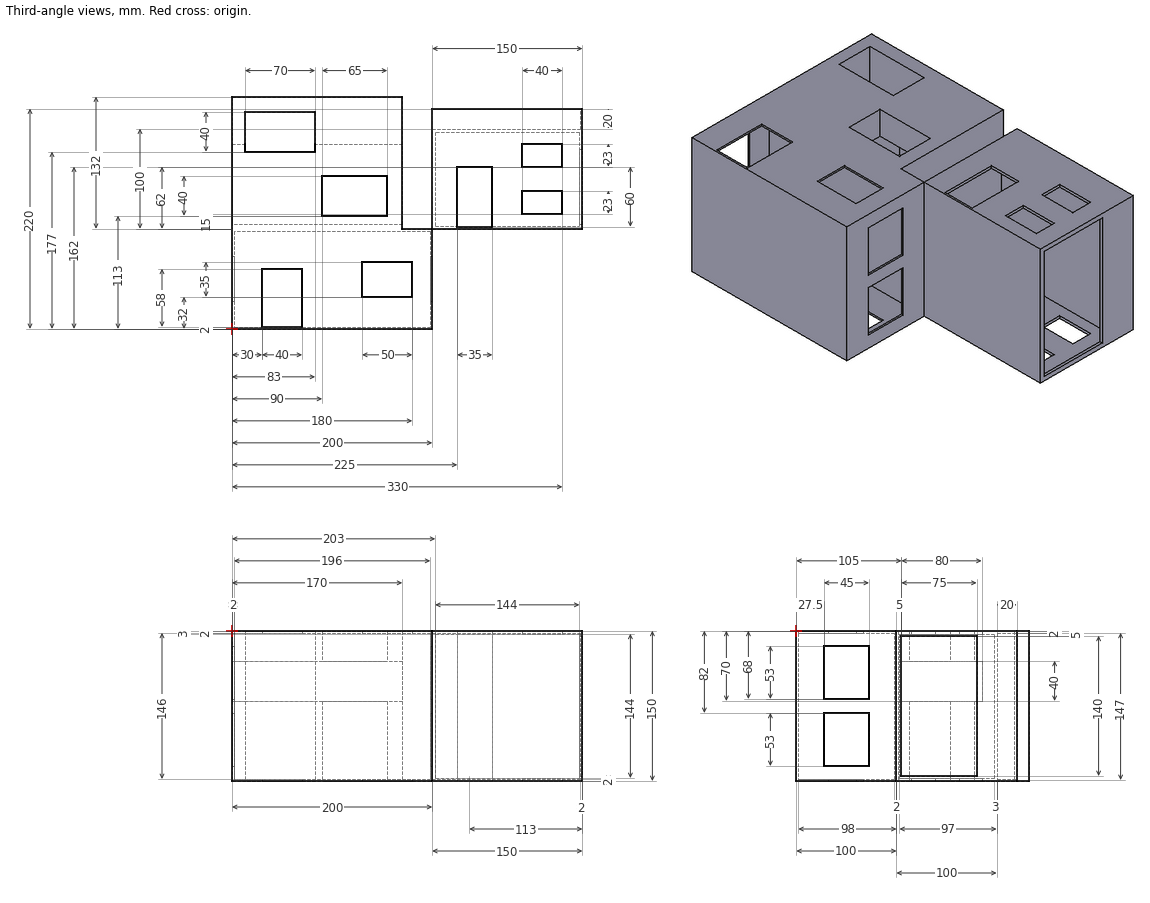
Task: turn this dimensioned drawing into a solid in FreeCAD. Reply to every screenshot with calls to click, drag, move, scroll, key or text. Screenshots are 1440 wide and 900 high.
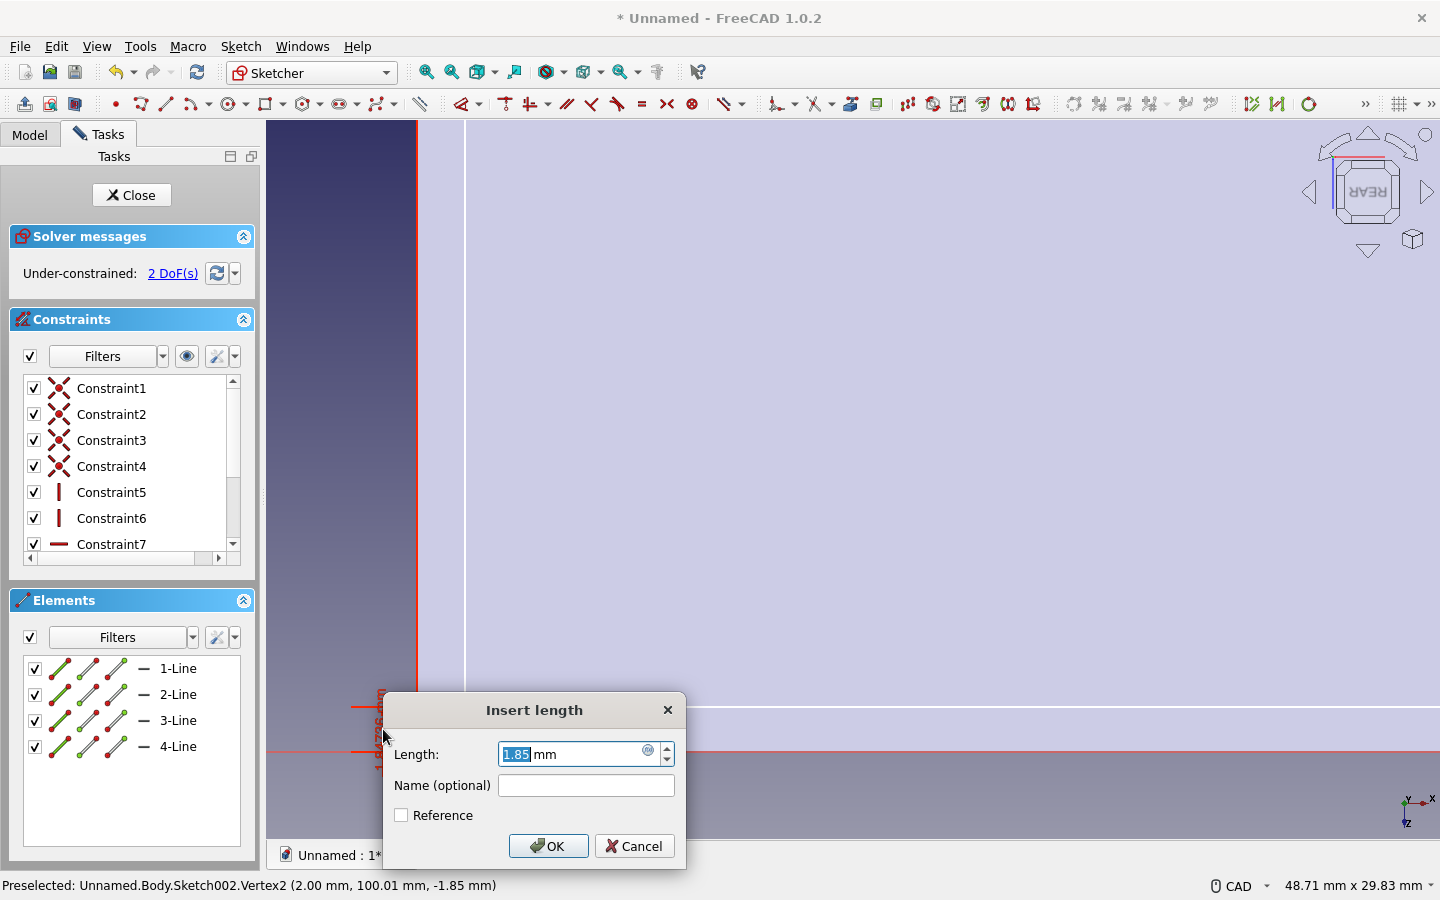
text(2)
key(Return)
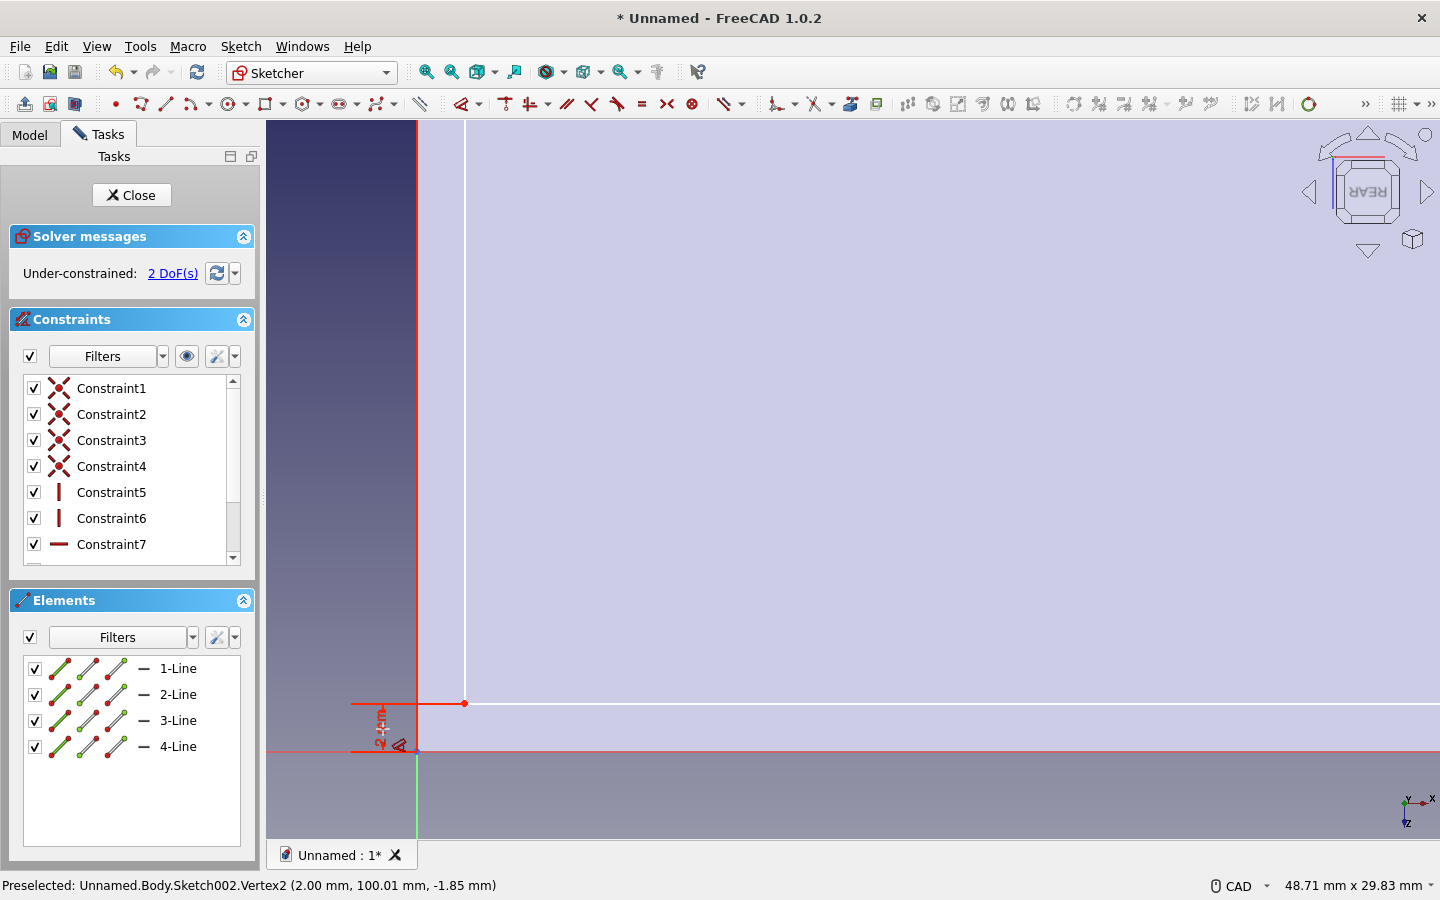
scroll(469, 716, down, 10)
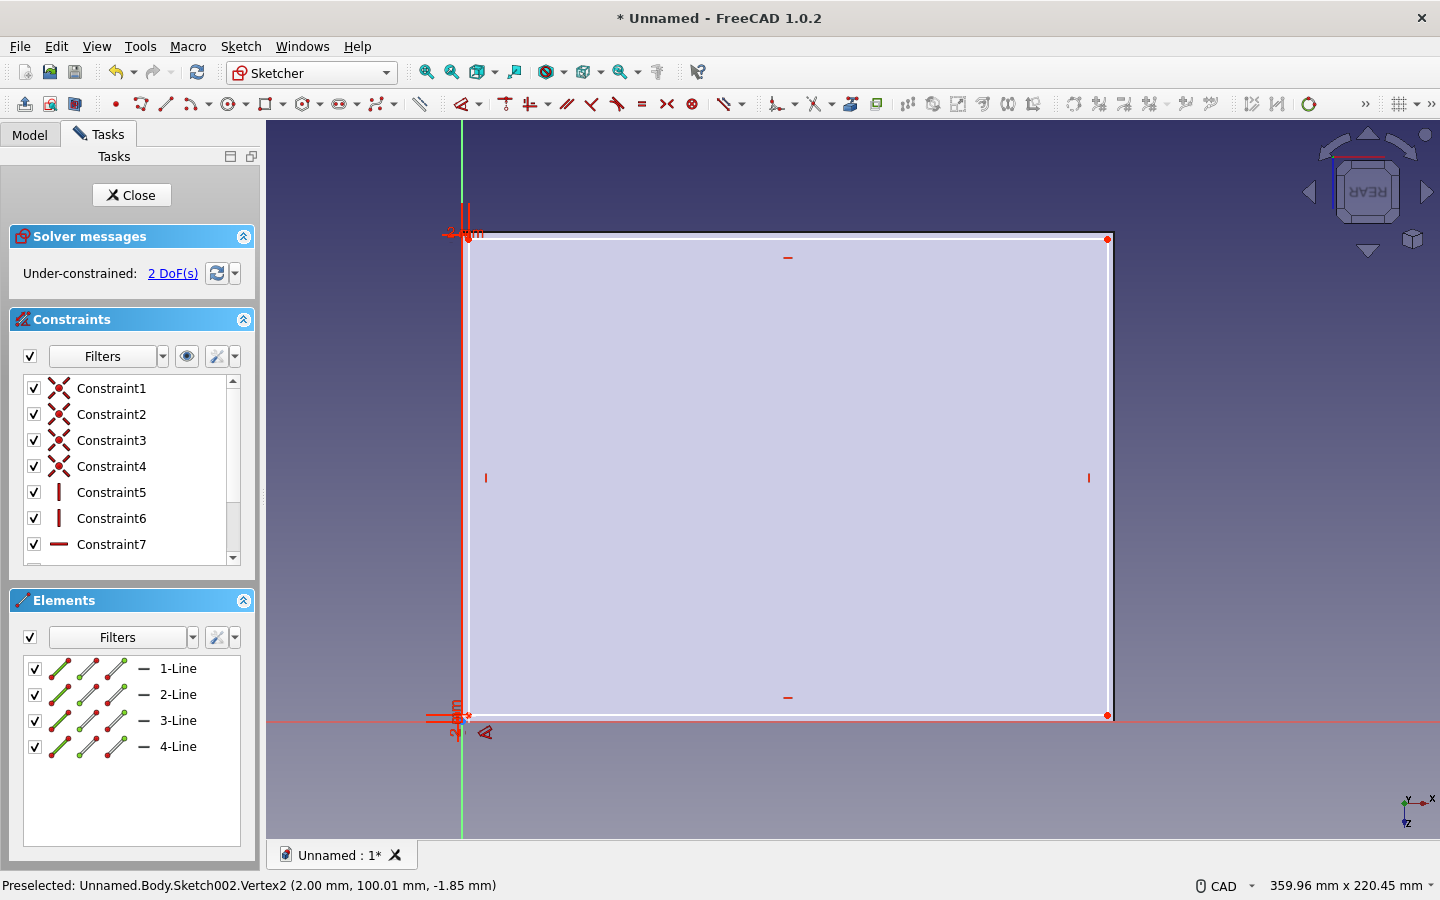
scroll(469, 382, up, 4)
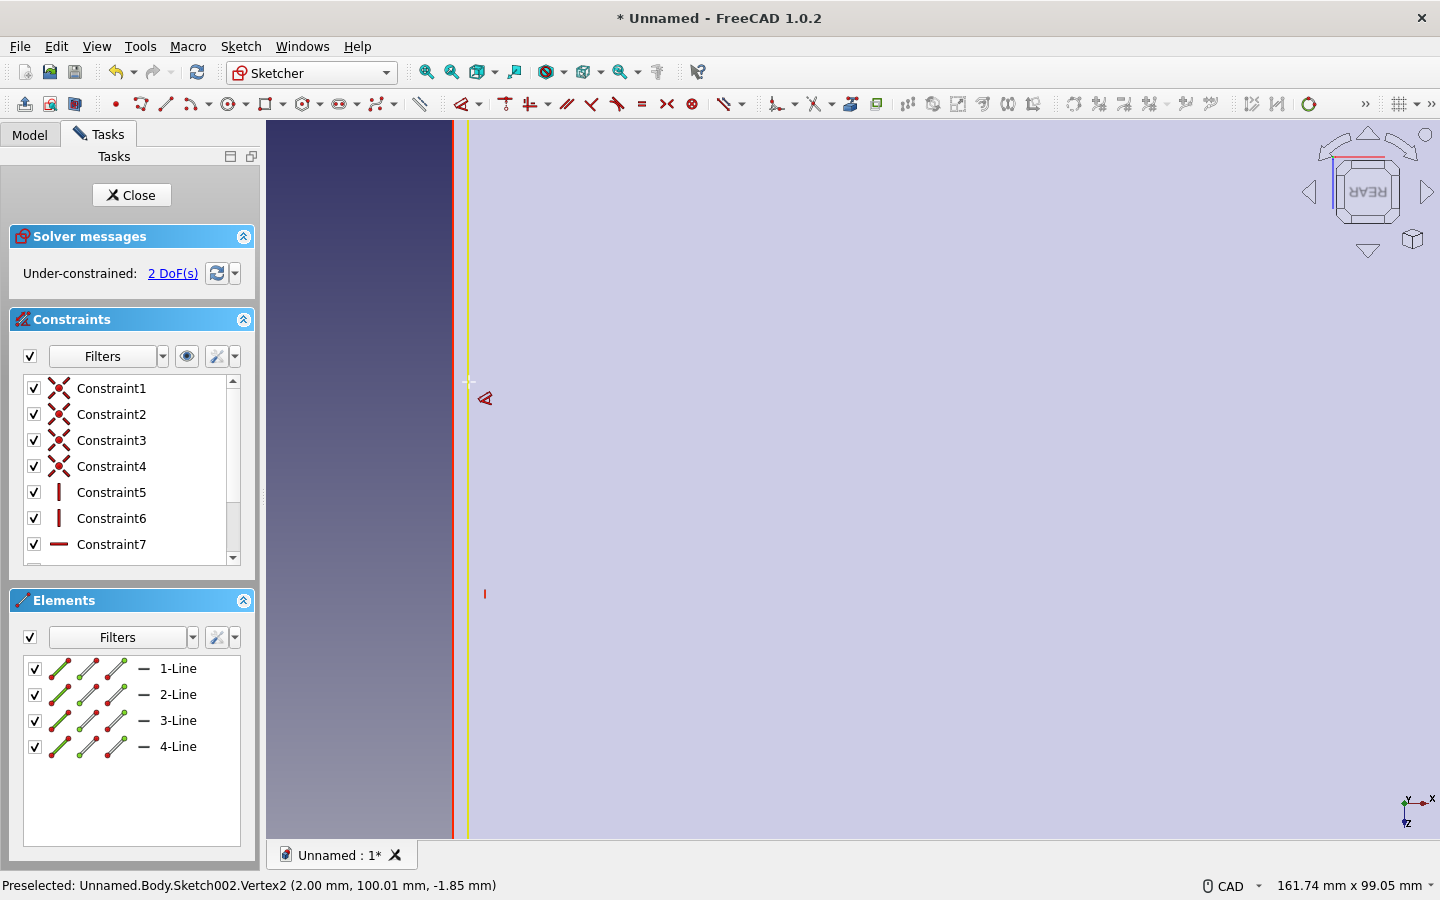
click(468, 381)
click(434, 480)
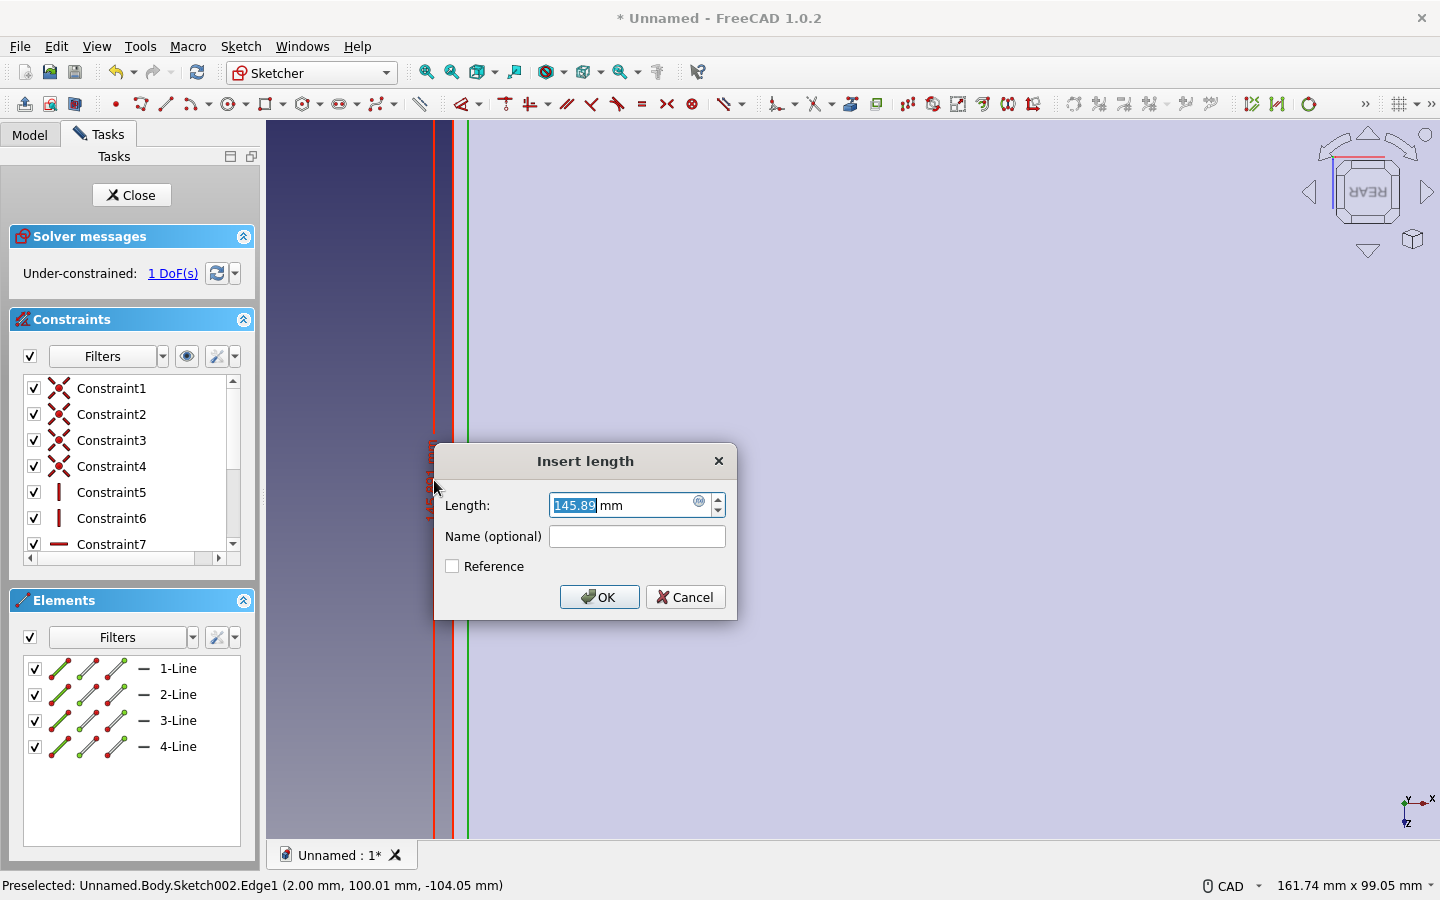
text(146)
key(Return)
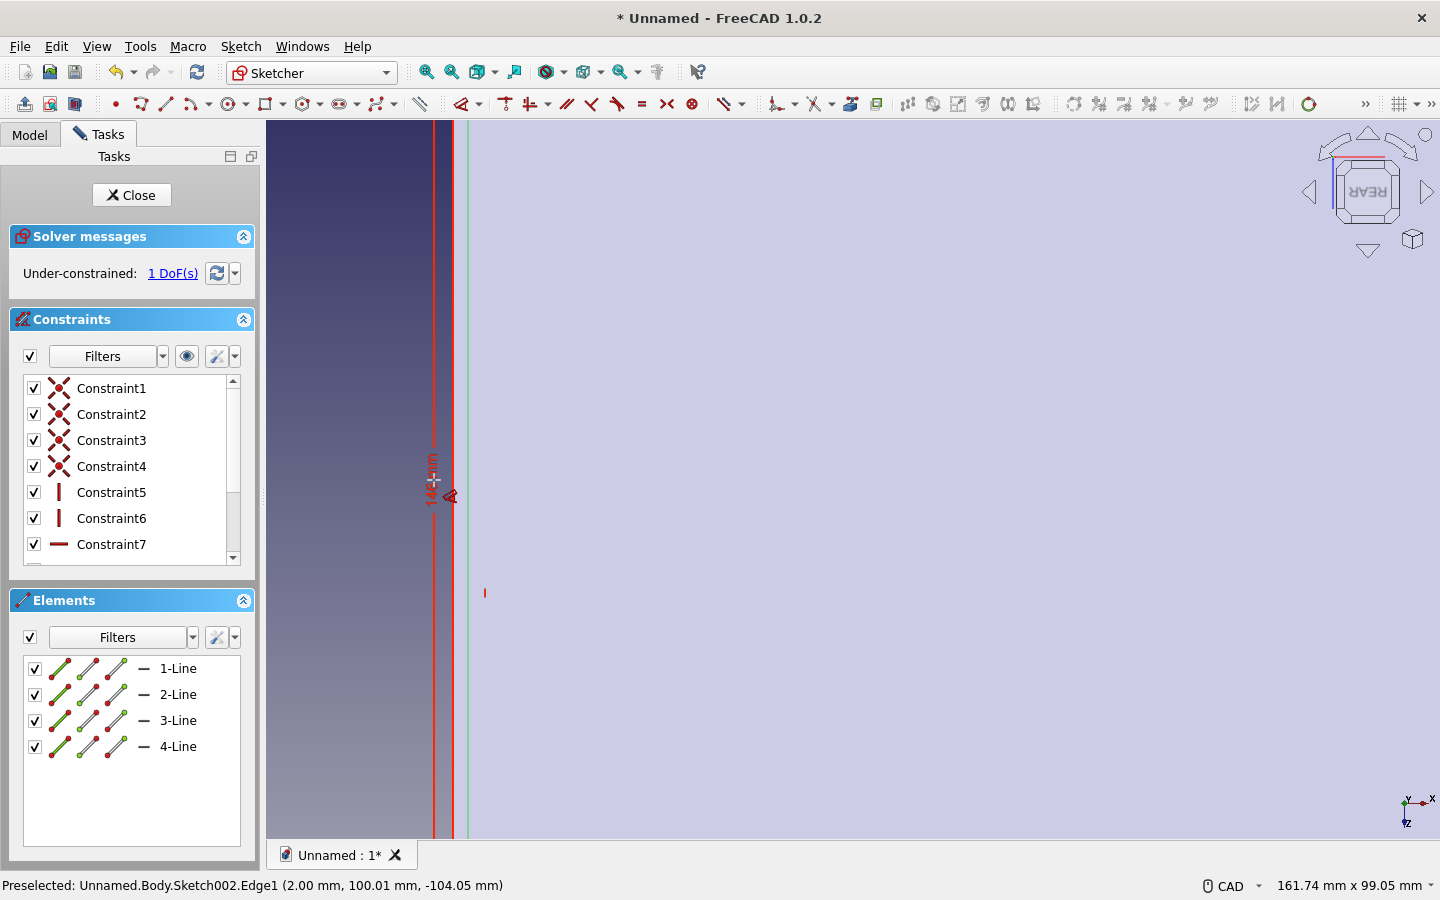
scroll(468, 381, down, 4)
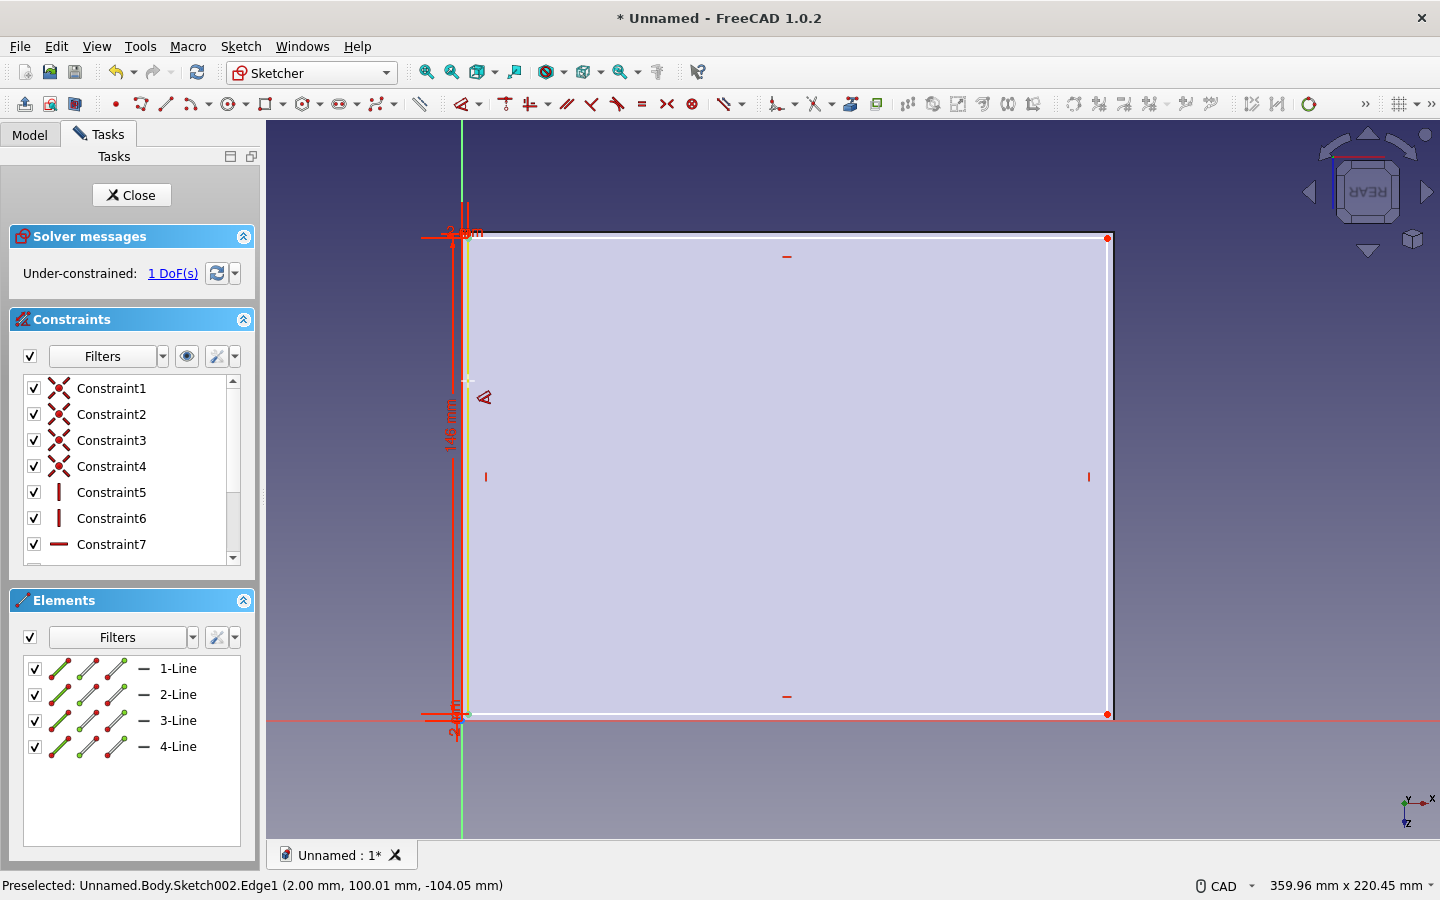
scroll(660, 714, up, 4)